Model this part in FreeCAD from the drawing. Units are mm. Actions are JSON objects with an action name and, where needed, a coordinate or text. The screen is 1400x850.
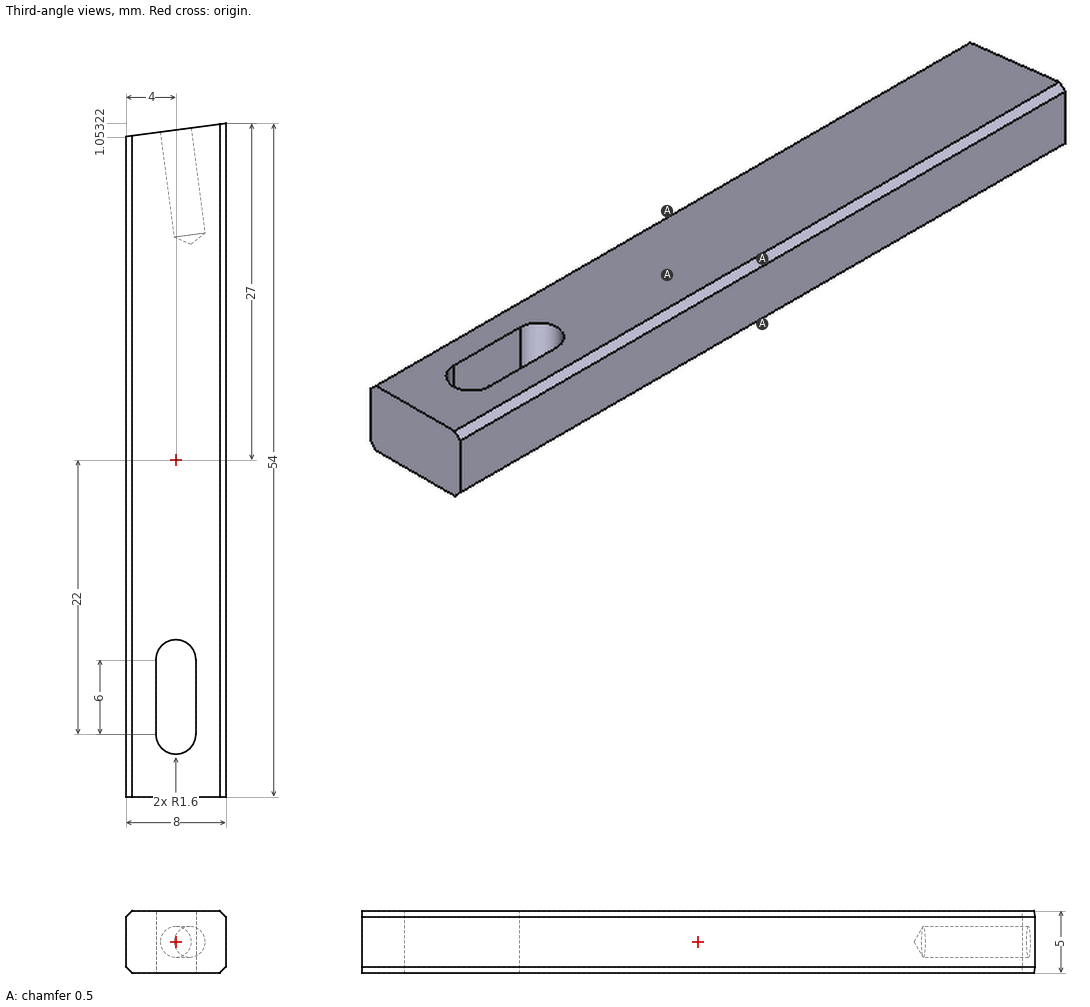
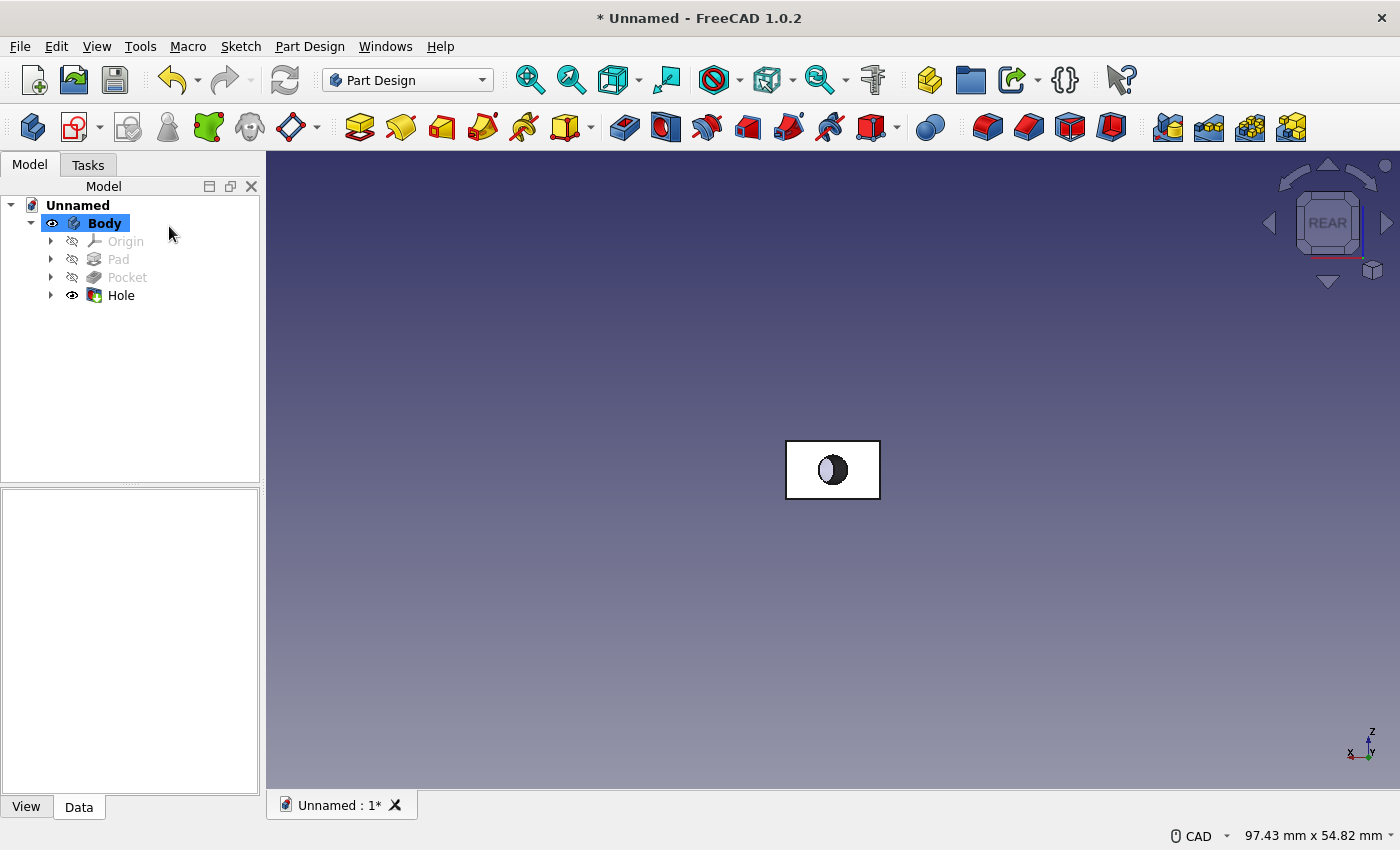
{"action": "key", "text": "0"}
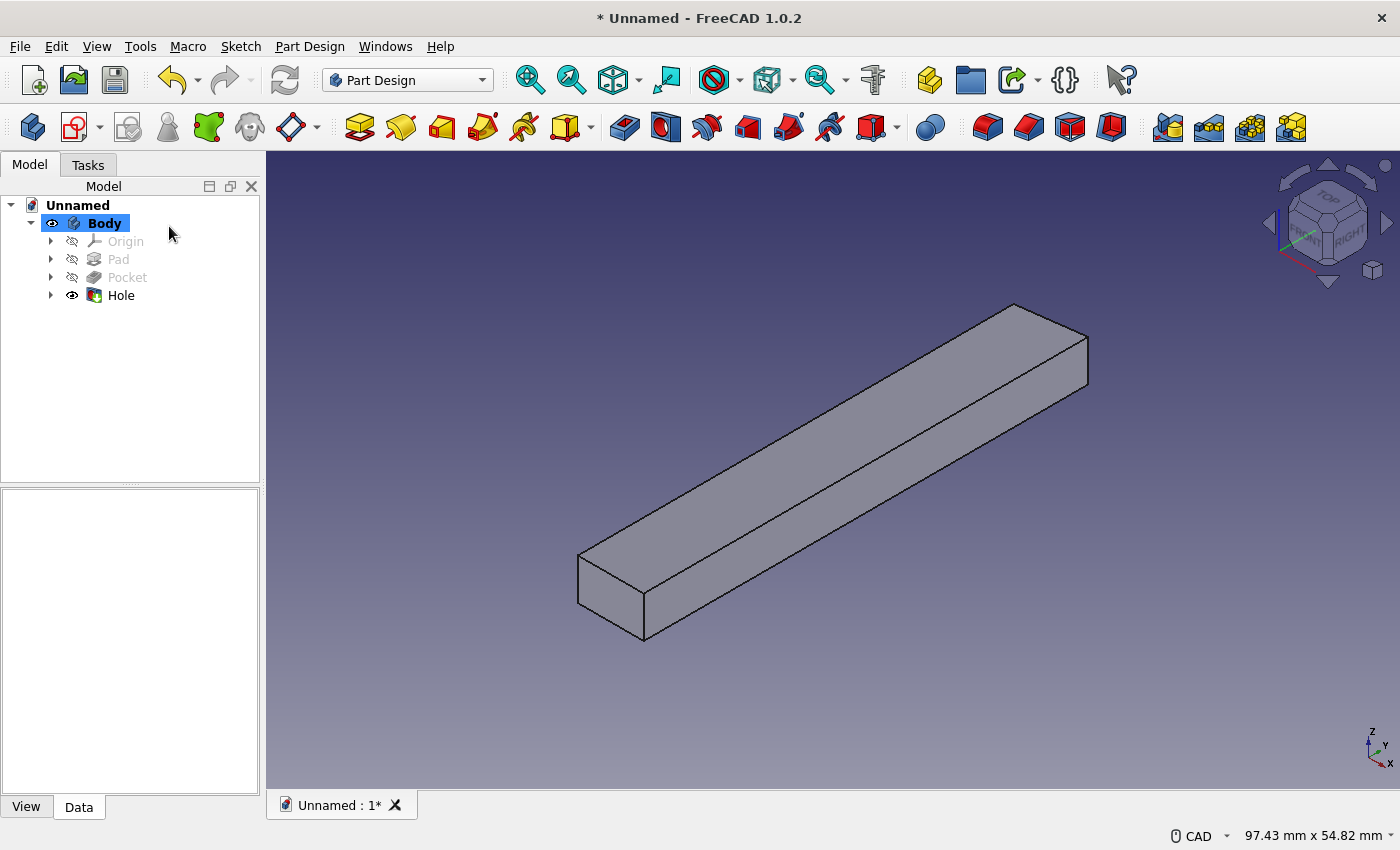
{"action": "left_click", "coordinate": [960, 372]}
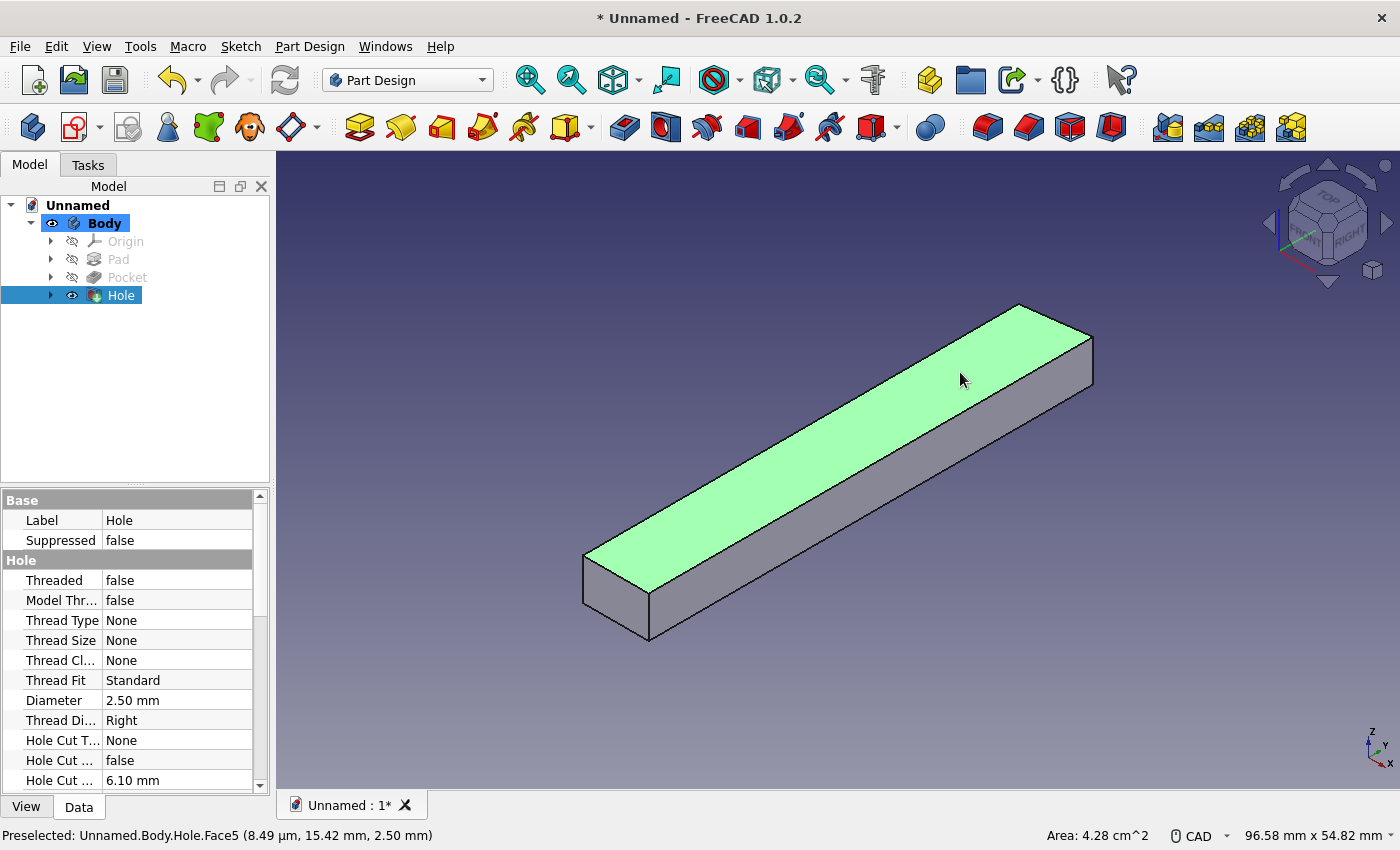
{"action": "left_click", "coordinate": [74, 128]}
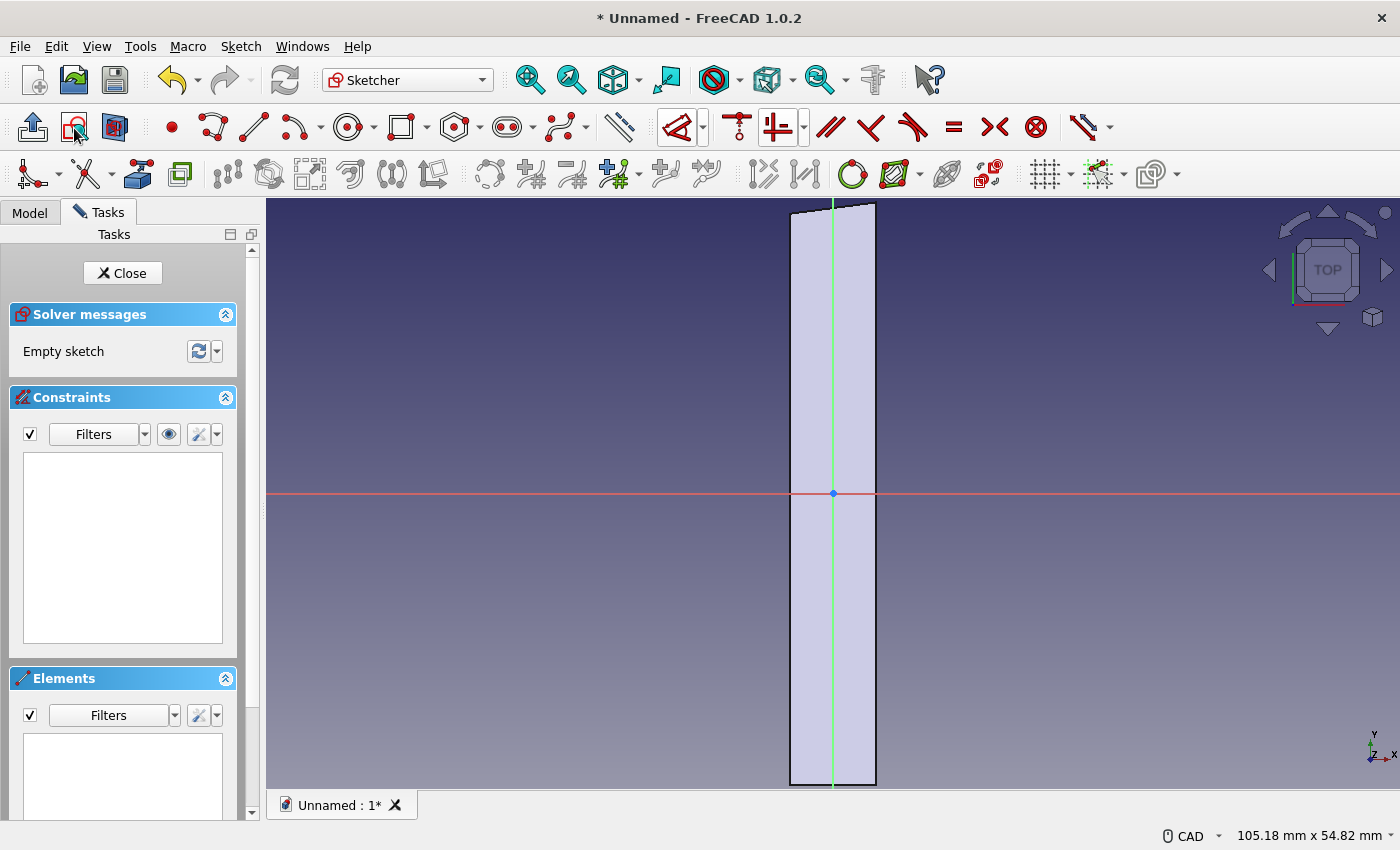
{"action": "scroll", "coordinate": [855, 761], "scroll_direction": "up", "scroll_amount": 7}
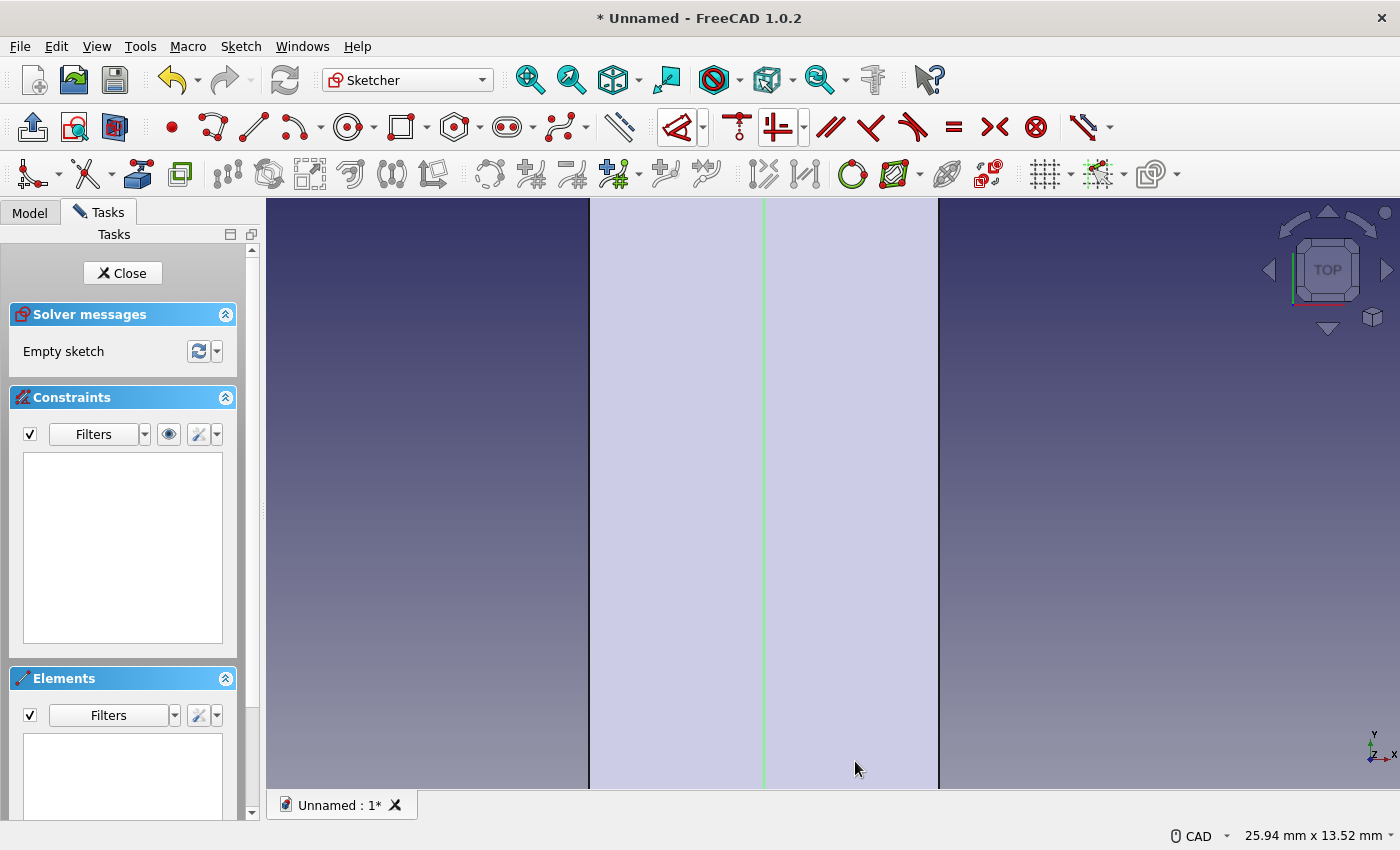
{"action": "key", "text": "g s"}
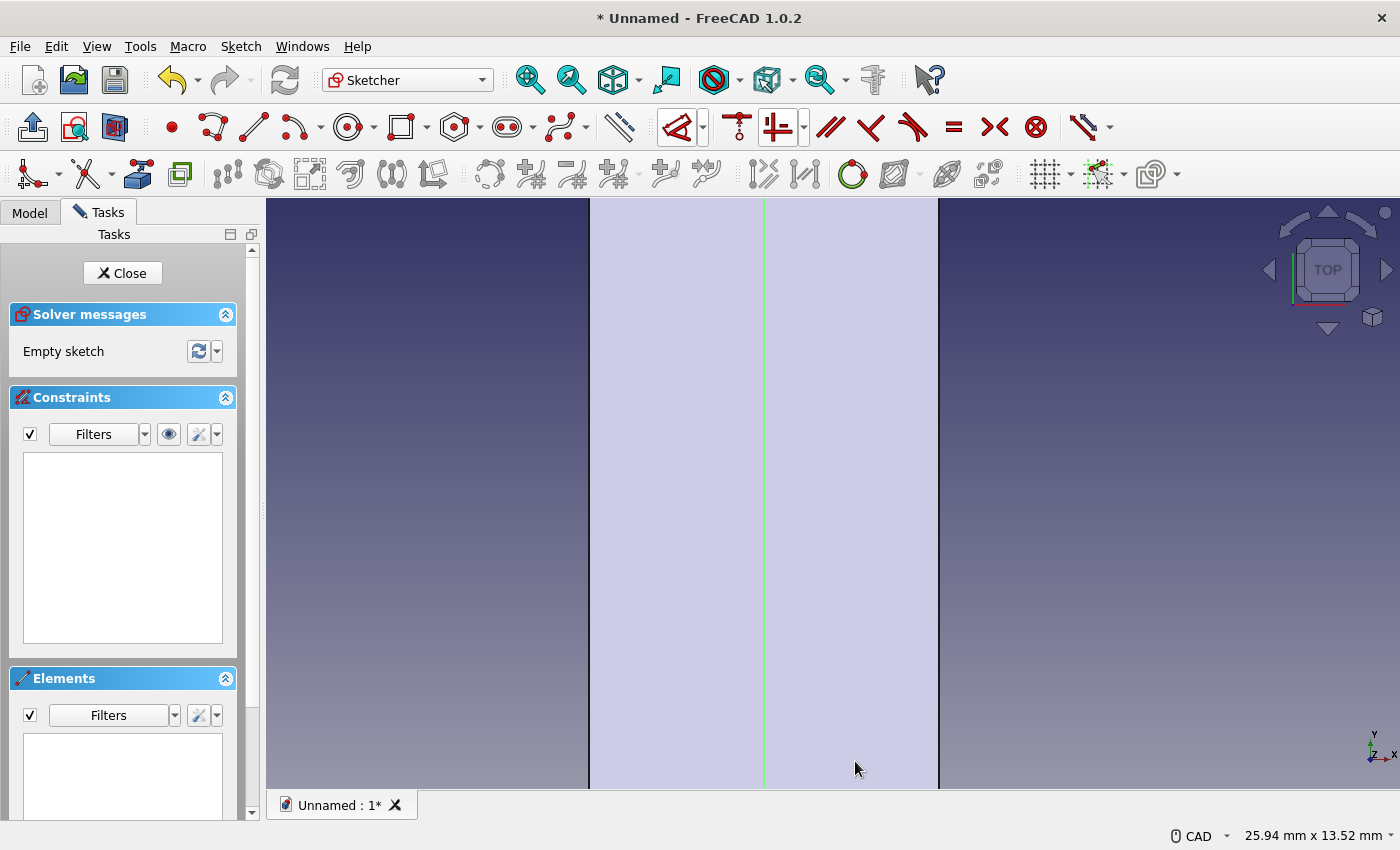
{"action": "left_click", "coordinate": [764, 635]}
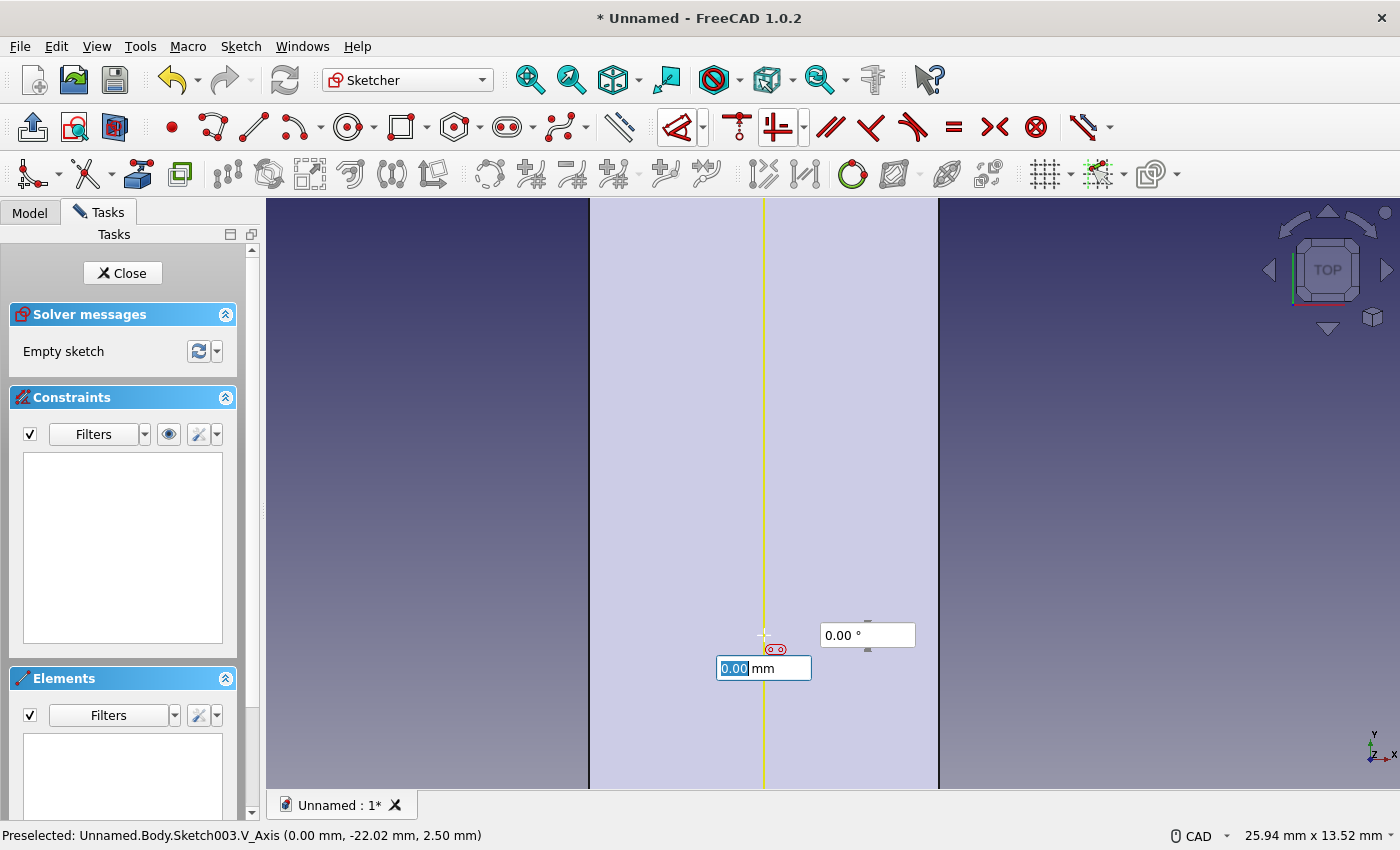
{"action": "left_click", "coordinate": [773, 373]}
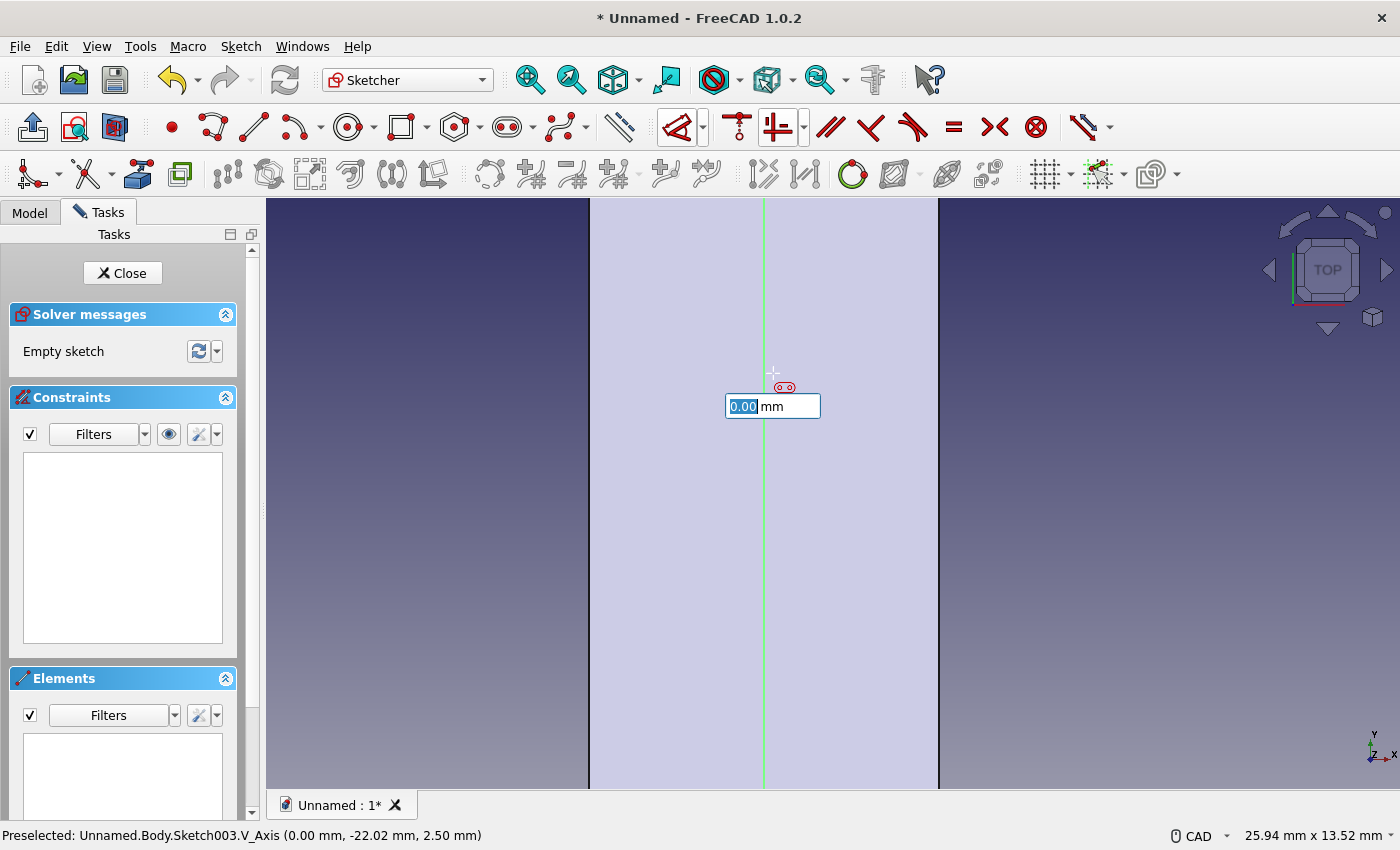
{"action": "left_click", "coordinate": [694, 504]}
{"action": "key", "text": "Escape"}